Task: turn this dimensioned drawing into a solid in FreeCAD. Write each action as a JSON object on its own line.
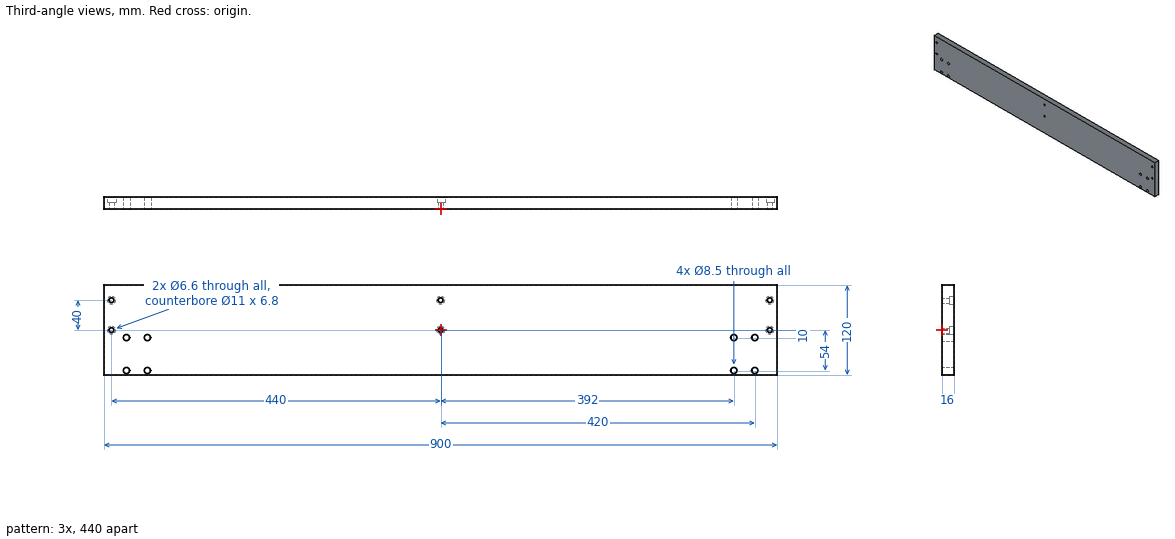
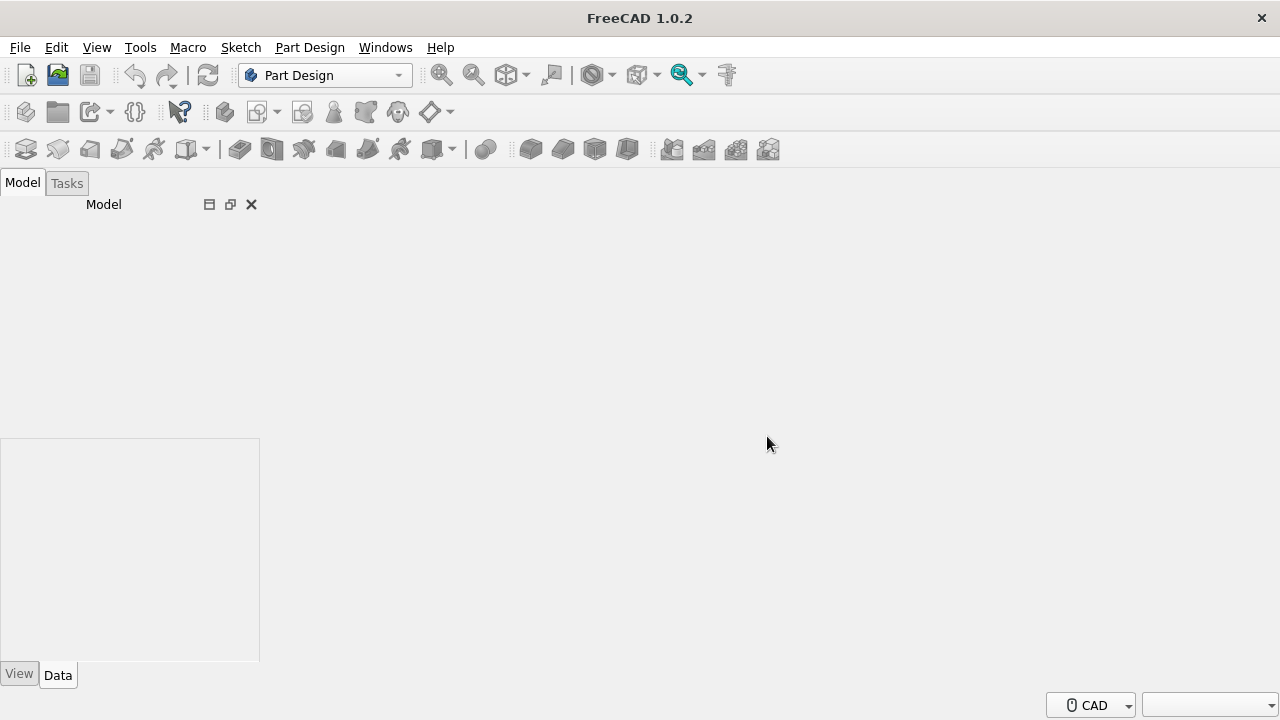
{"action": "key", "text": "ctrl+n"}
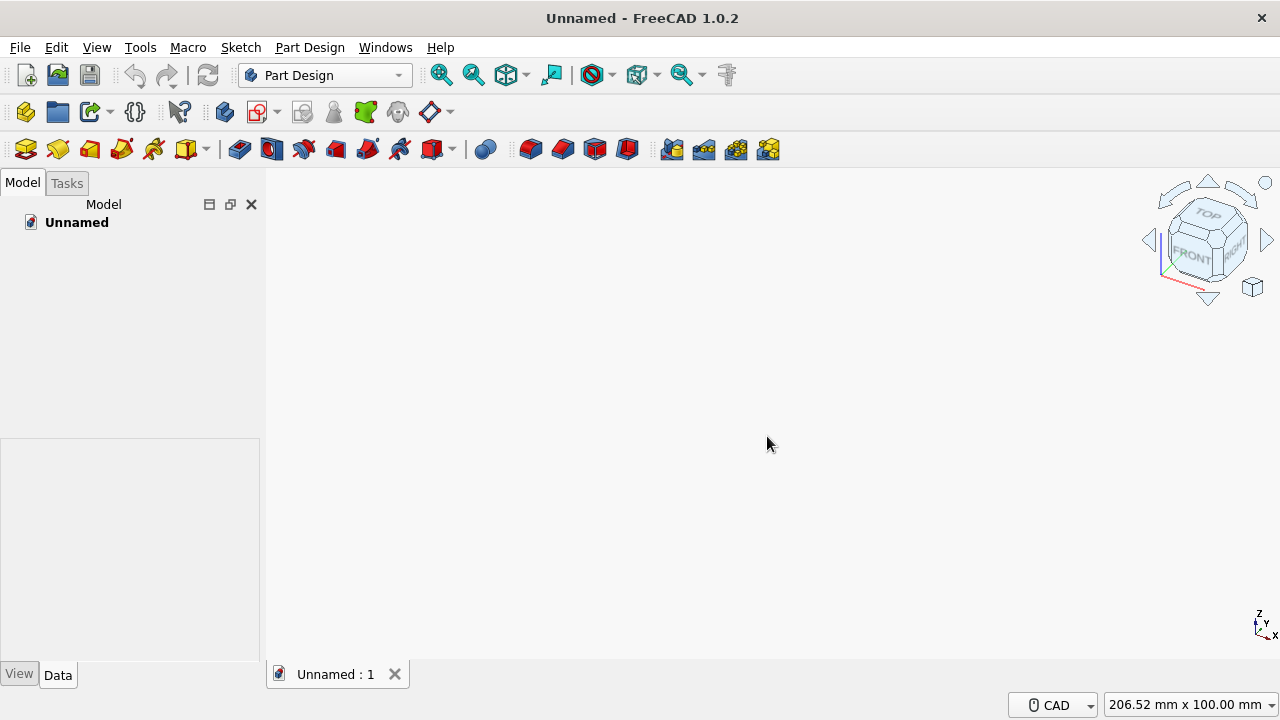
{"action": "left_click", "coordinate": [258, 112]}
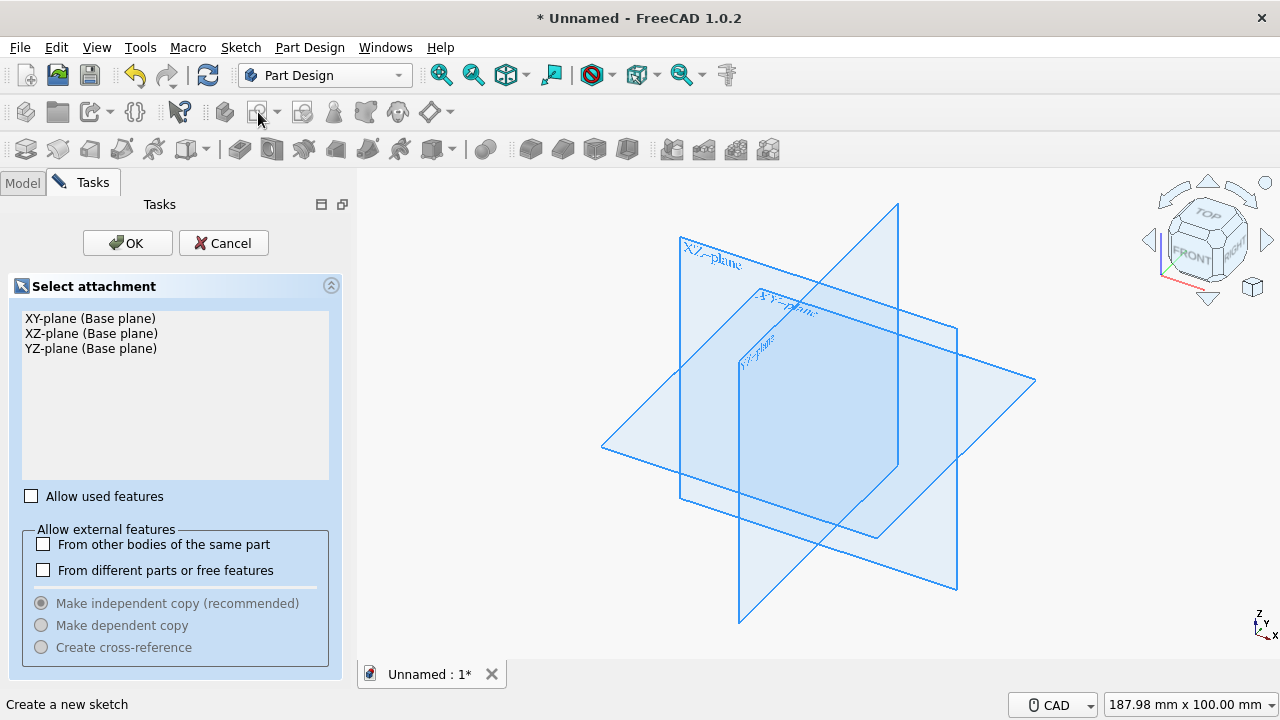
{"action": "left_click", "coordinate": [82, 334]}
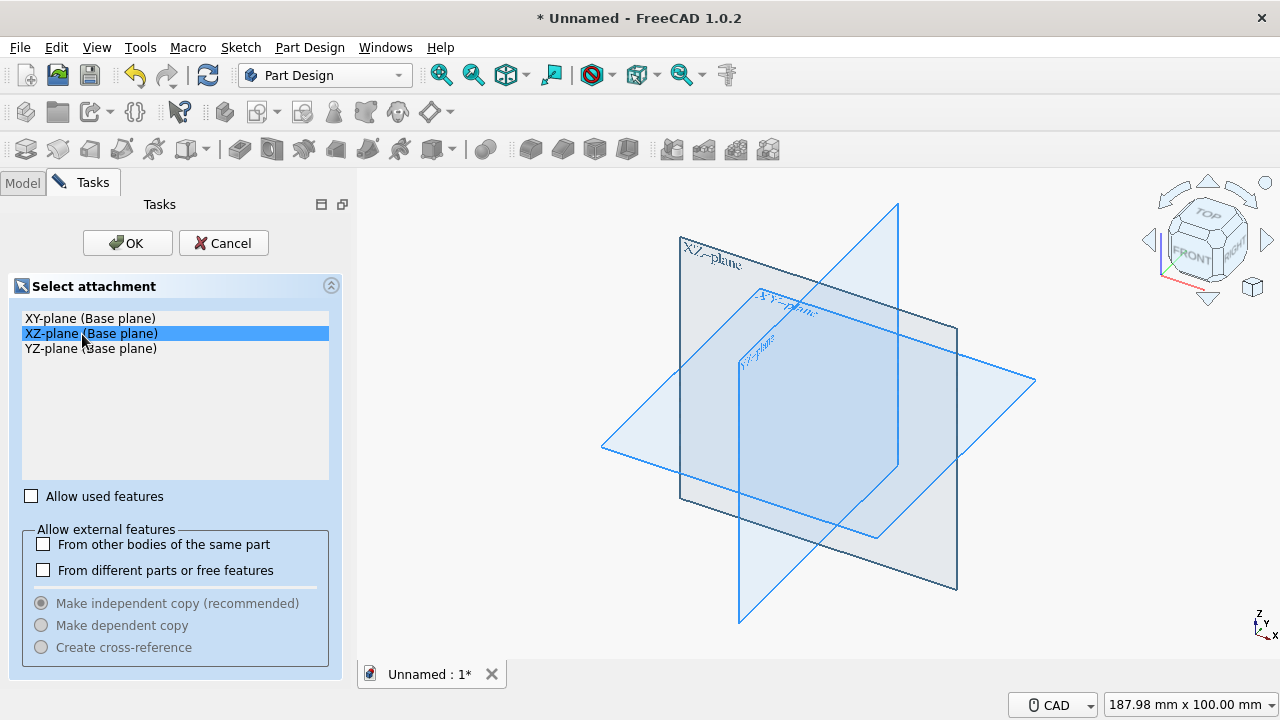
{"action": "left_click", "coordinate": [128, 243]}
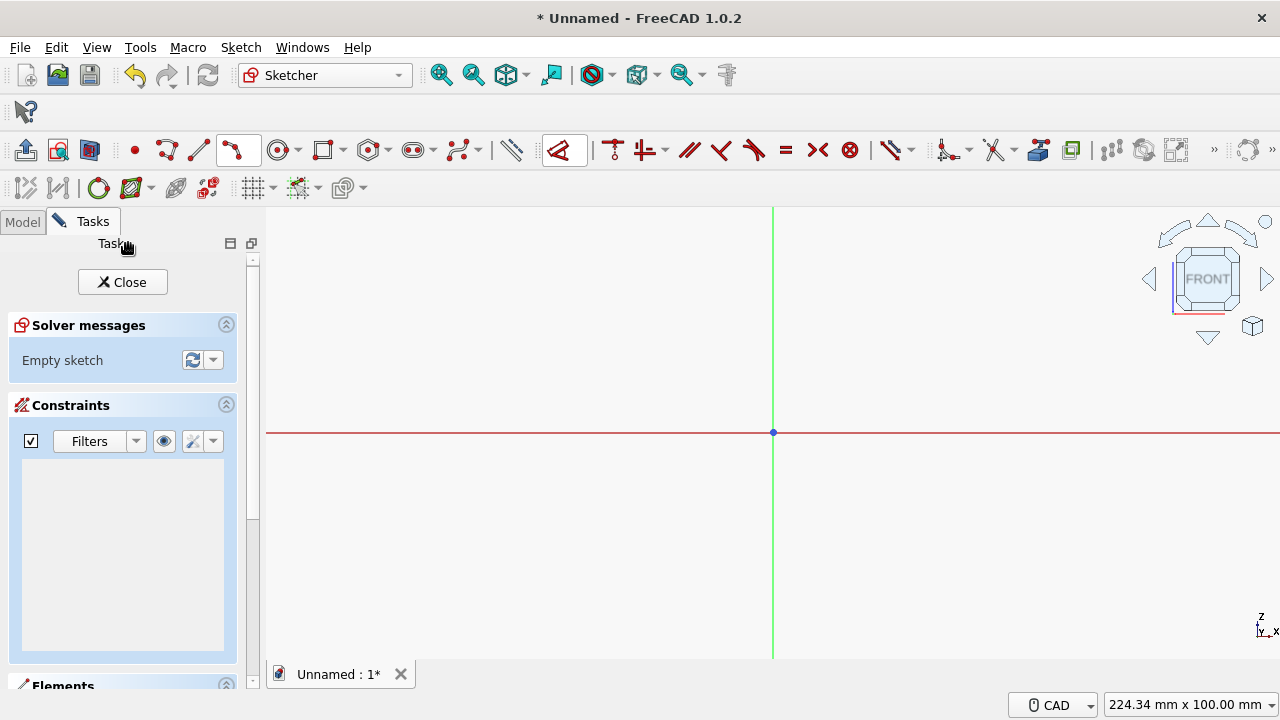
{"action": "scroll", "coordinate": [694, 433], "scroll_direction": "down", "scroll_amount": 10}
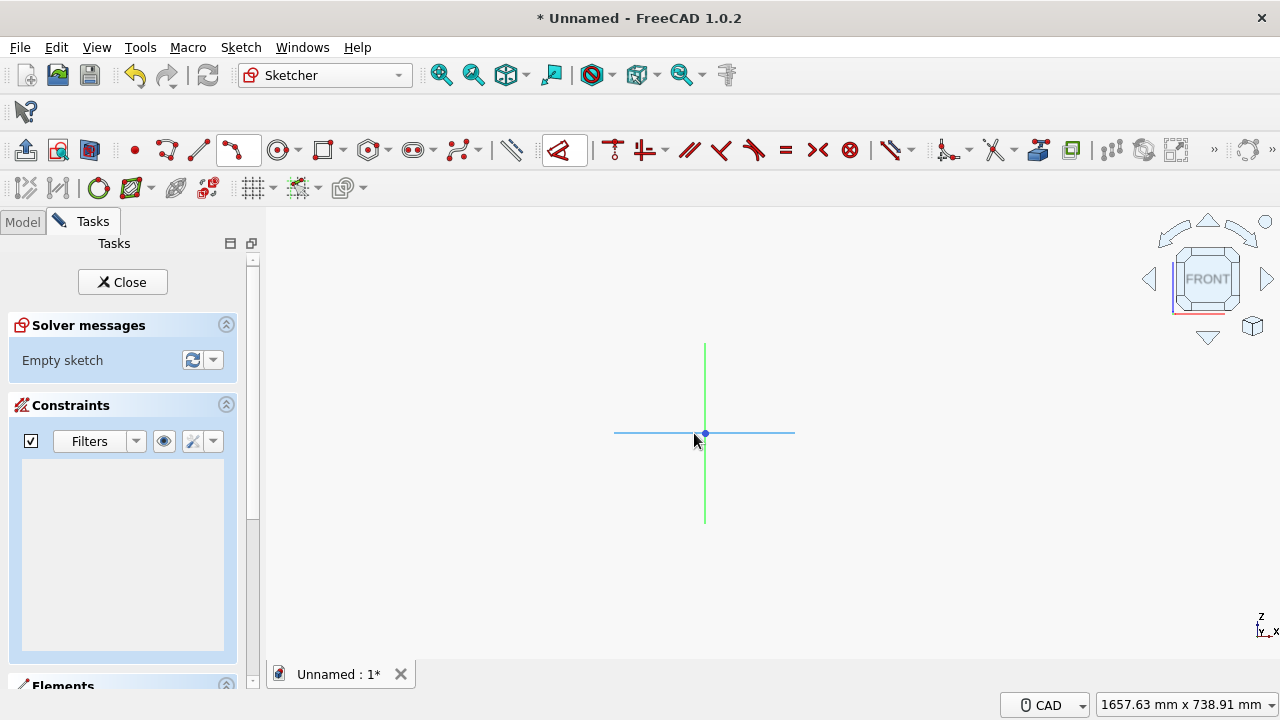
{"action": "key", "text": "g v"}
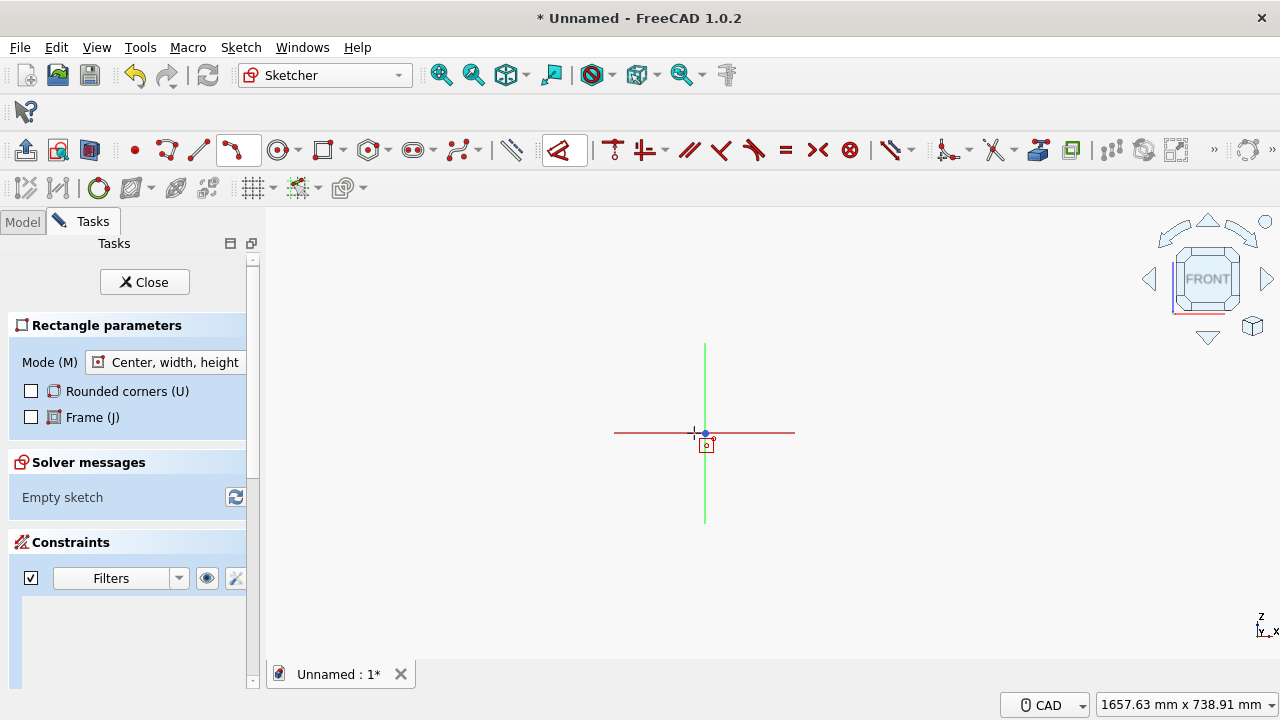
{"action": "left_click", "coordinate": [705, 433]}
{"action": "mouse_move", "coordinate": [980, 397]}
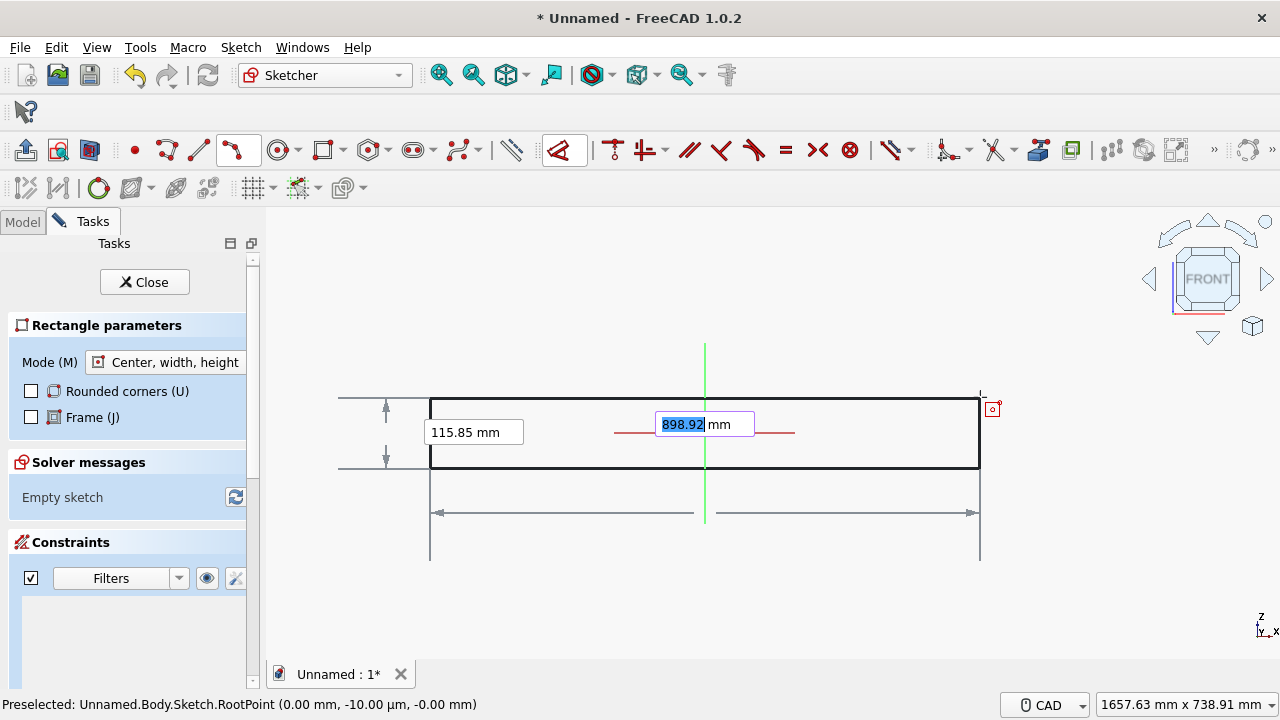
{"action": "type", "text": "900"}
{"action": "key", "text": "Tab"}
{"action": "type", "text": "120"}
{"action": "key", "text": "Return"}
{"action": "key", "text": "Escape"}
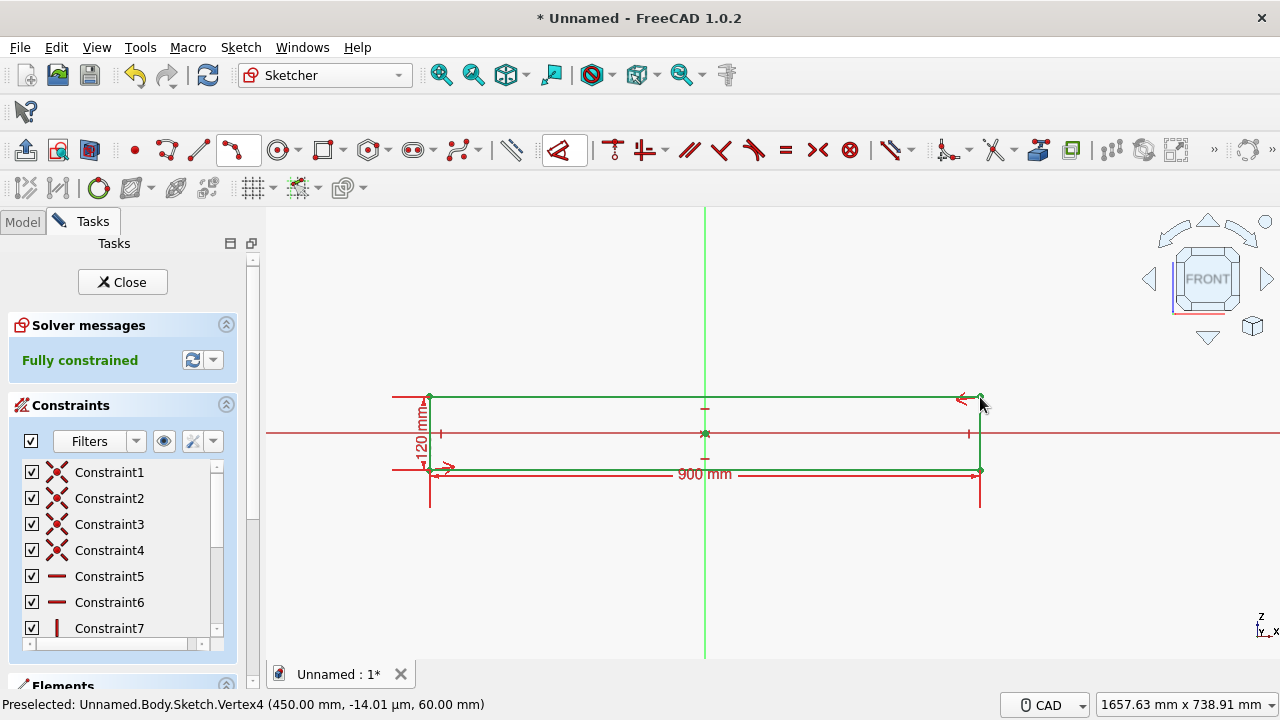
{"action": "left_click", "coordinate": [123, 282]}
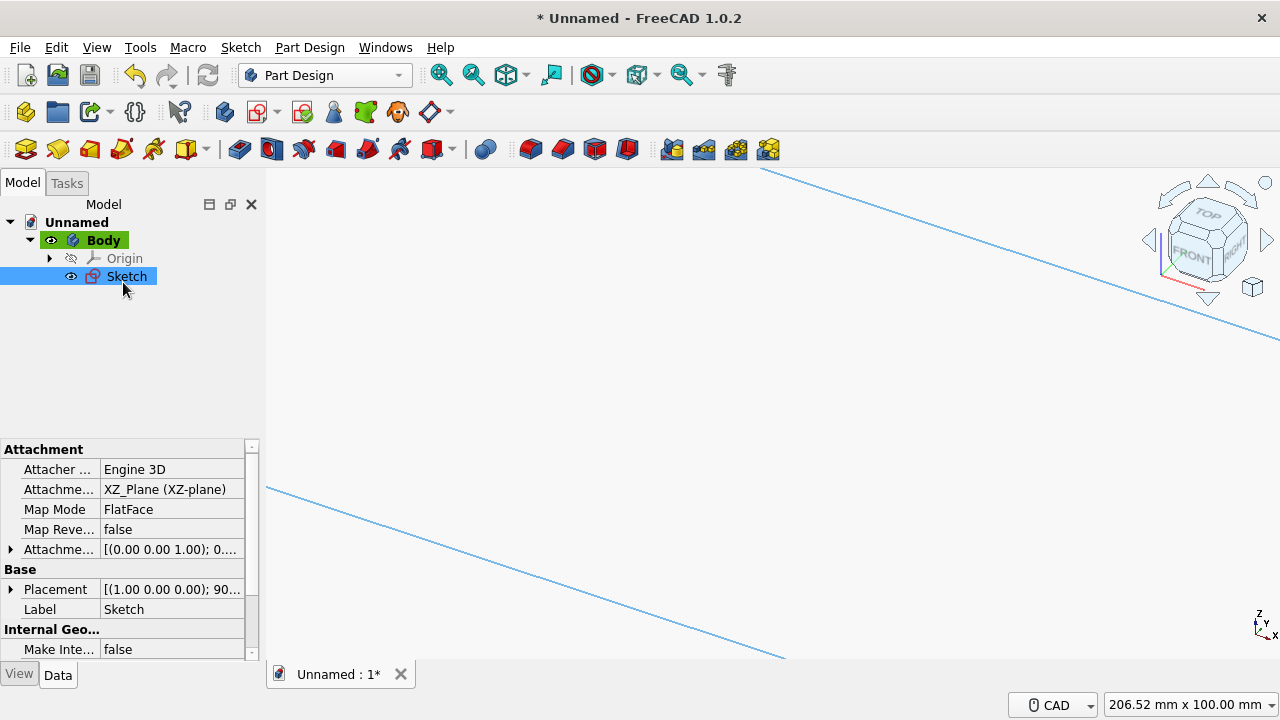
{"action": "left_click", "coordinate": [26, 150]}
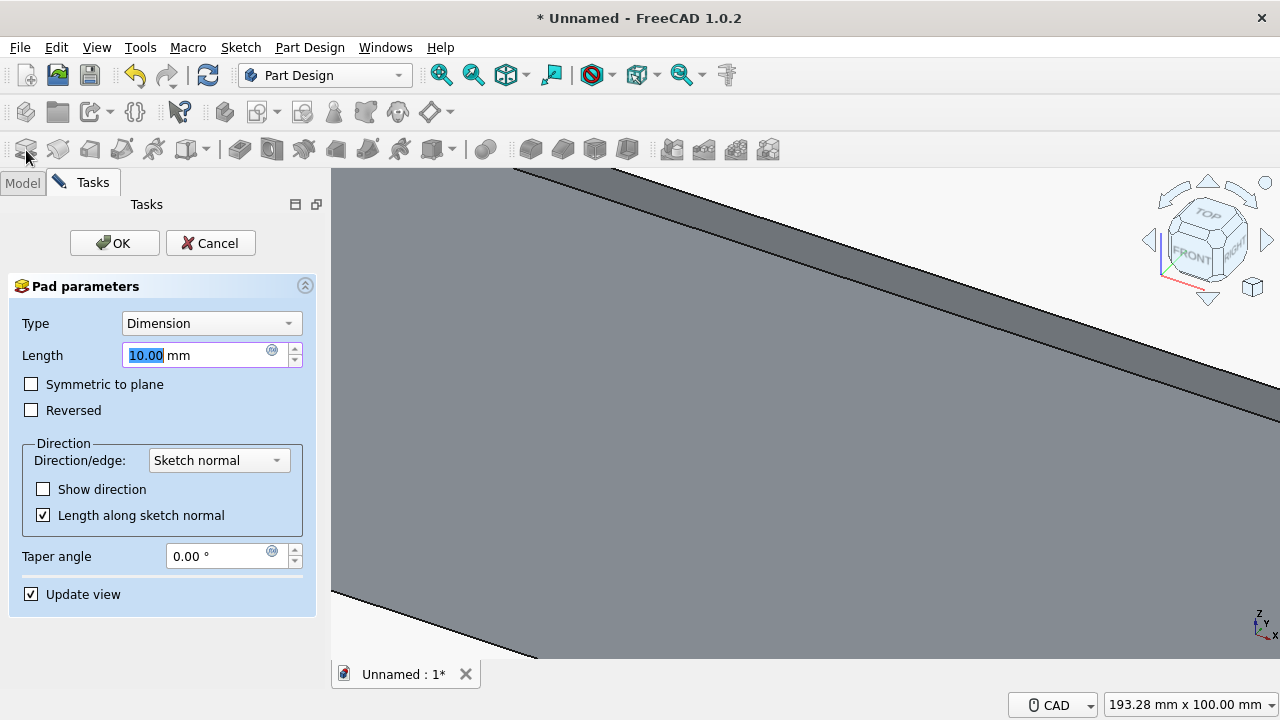
{"action": "type", "text": "16"}
{"action": "key", "text": "Tab"}